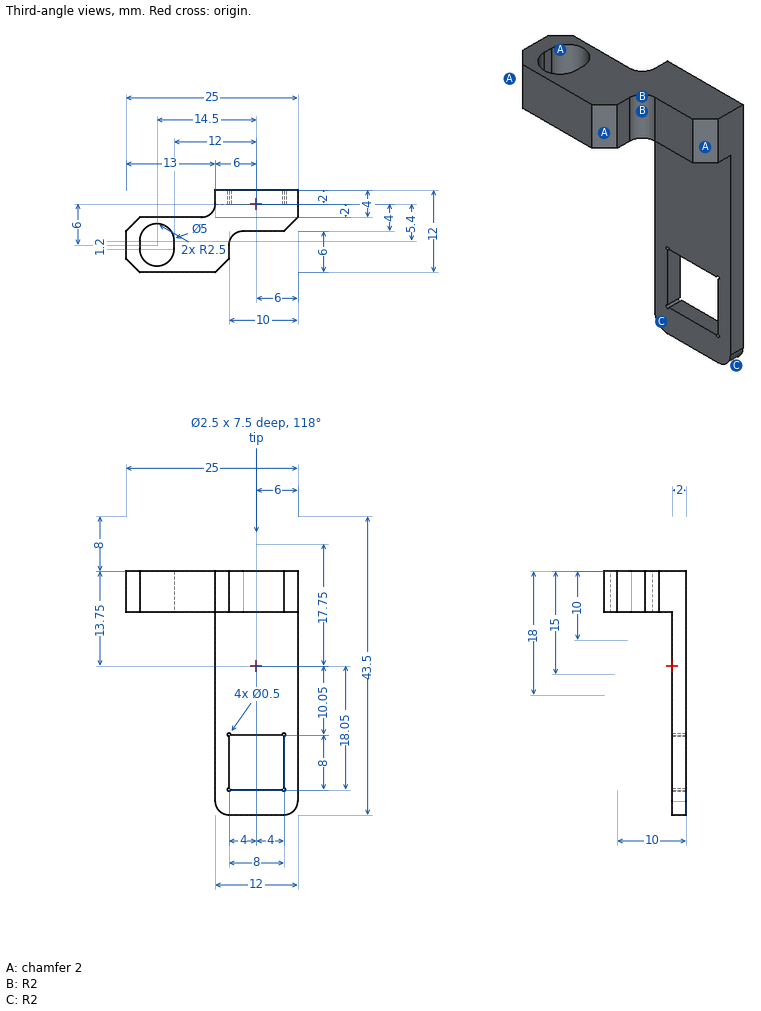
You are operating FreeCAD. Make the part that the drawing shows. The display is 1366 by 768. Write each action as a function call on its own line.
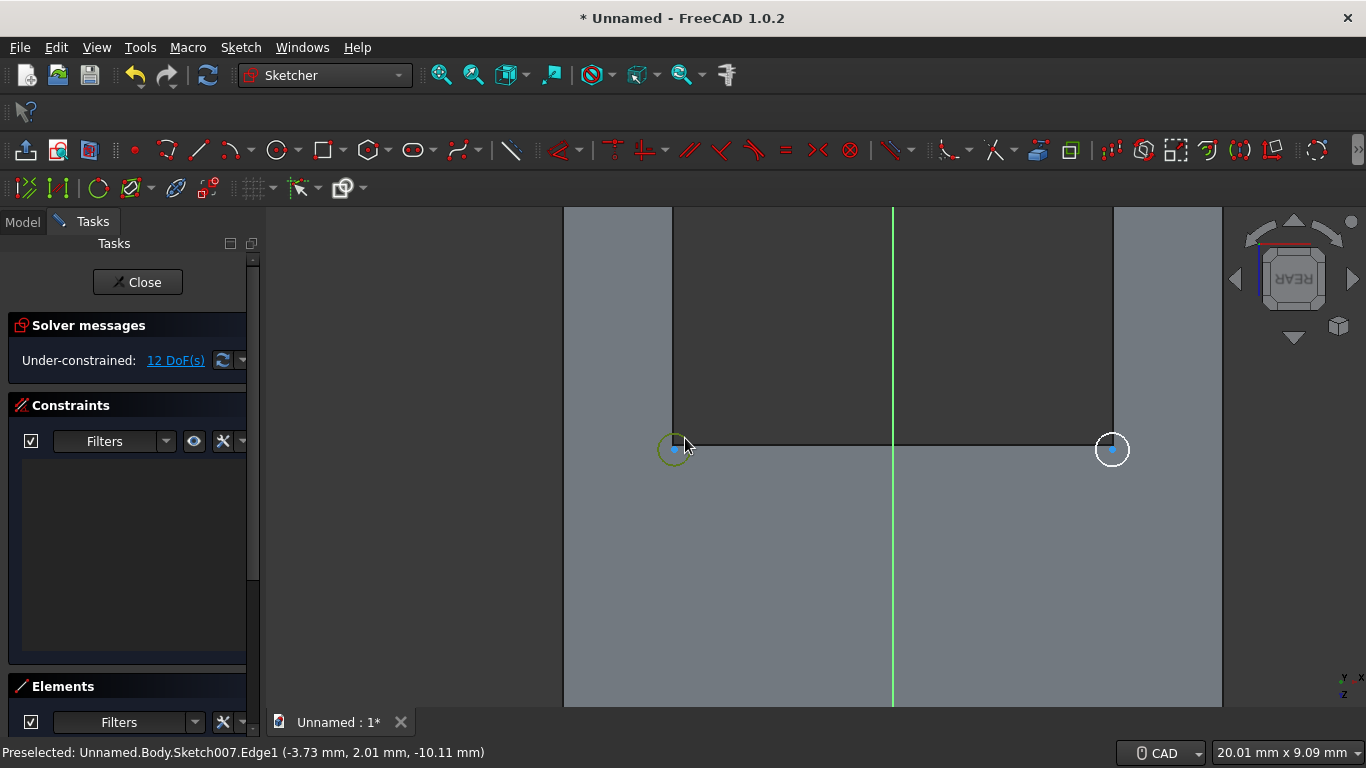
click(1124, 438)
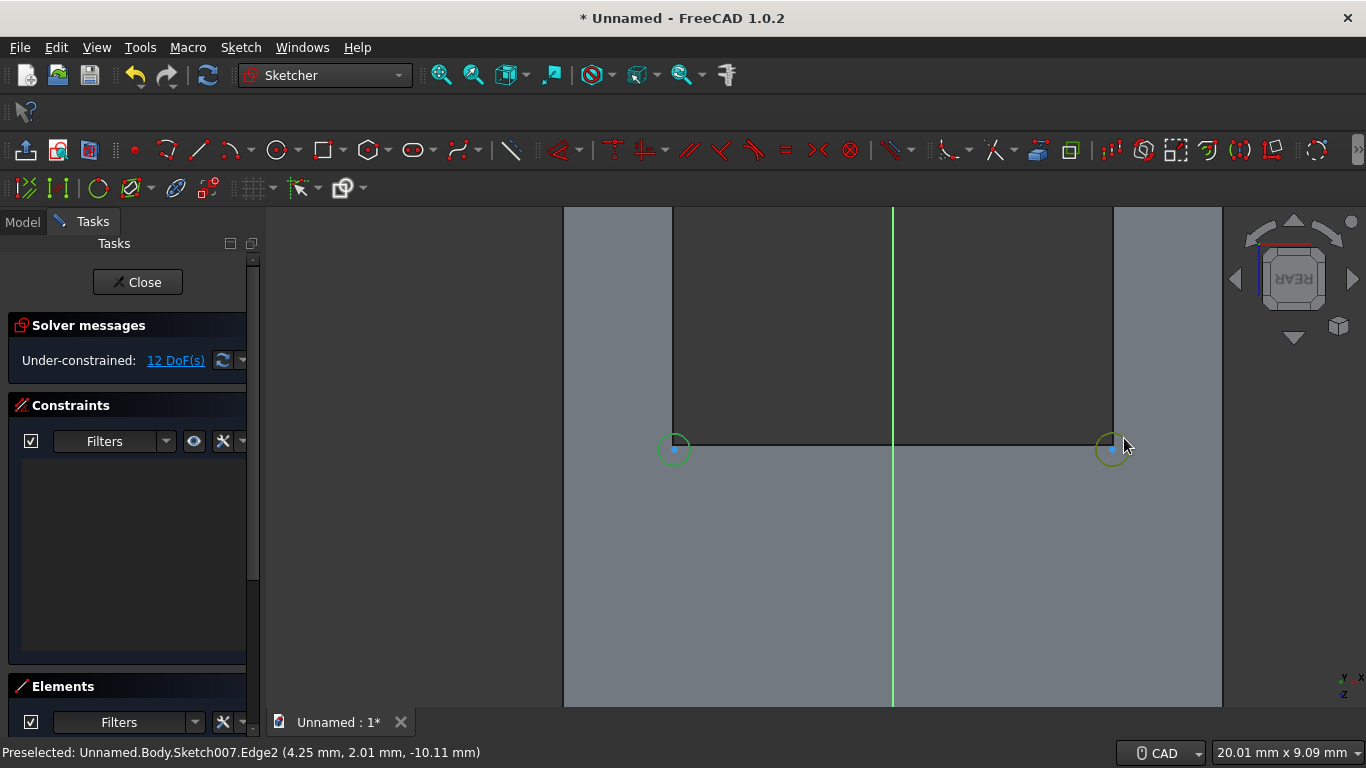
scroll(685, 441, down, 6)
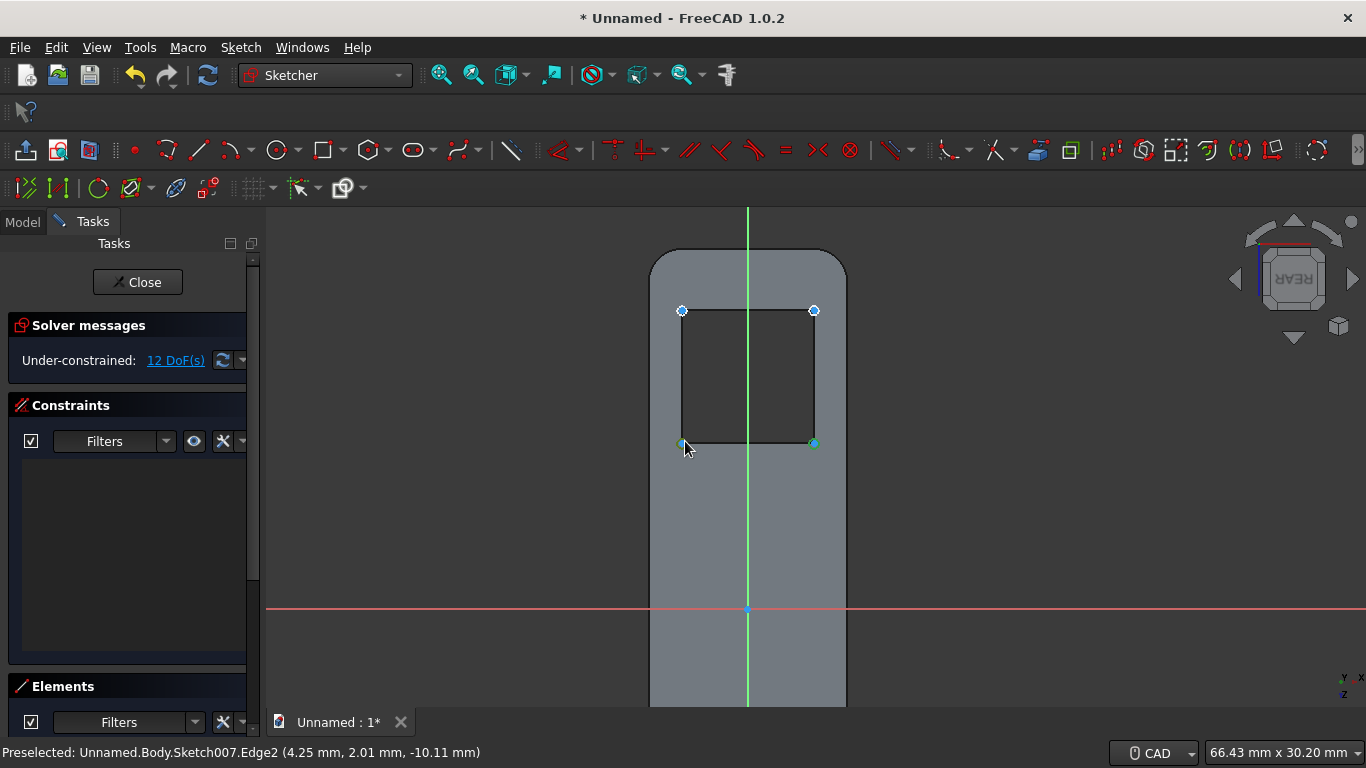
scroll(685, 308, up, 6)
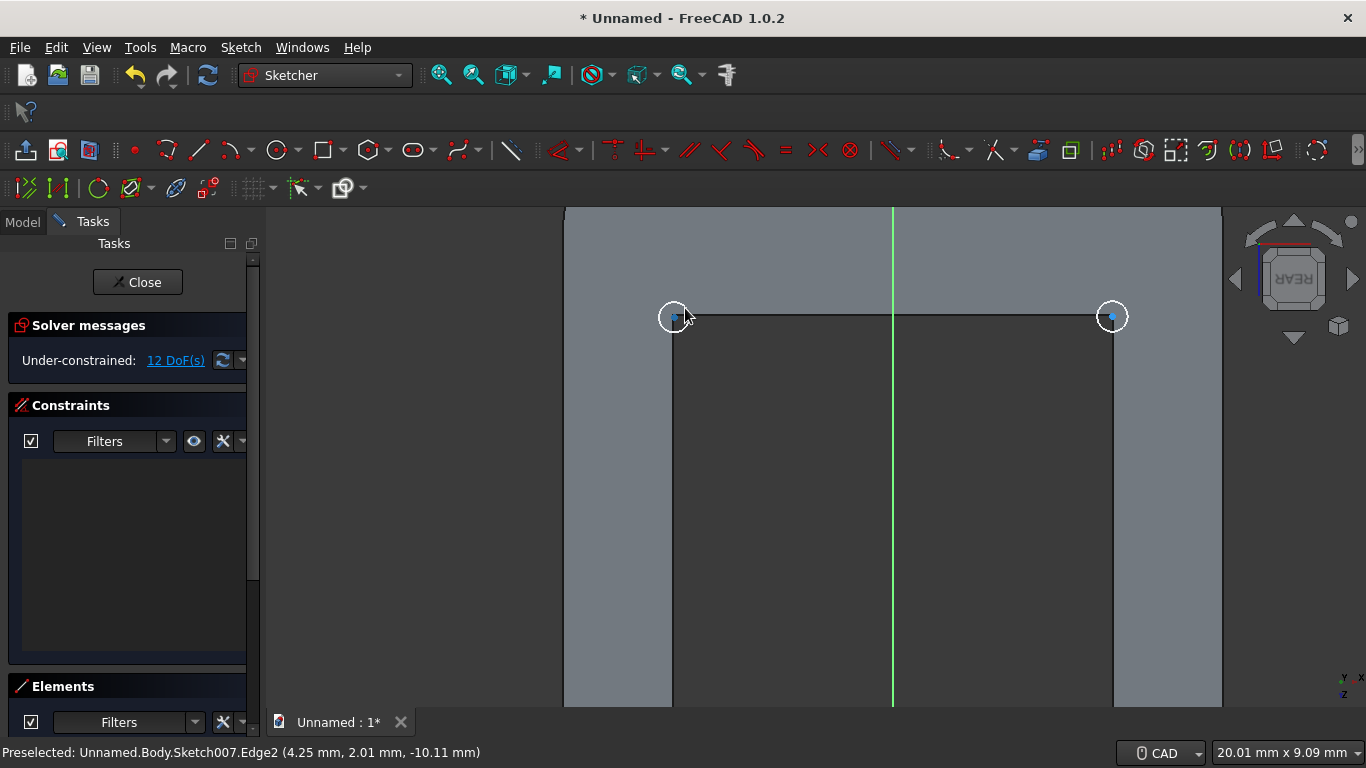
click(685, 307)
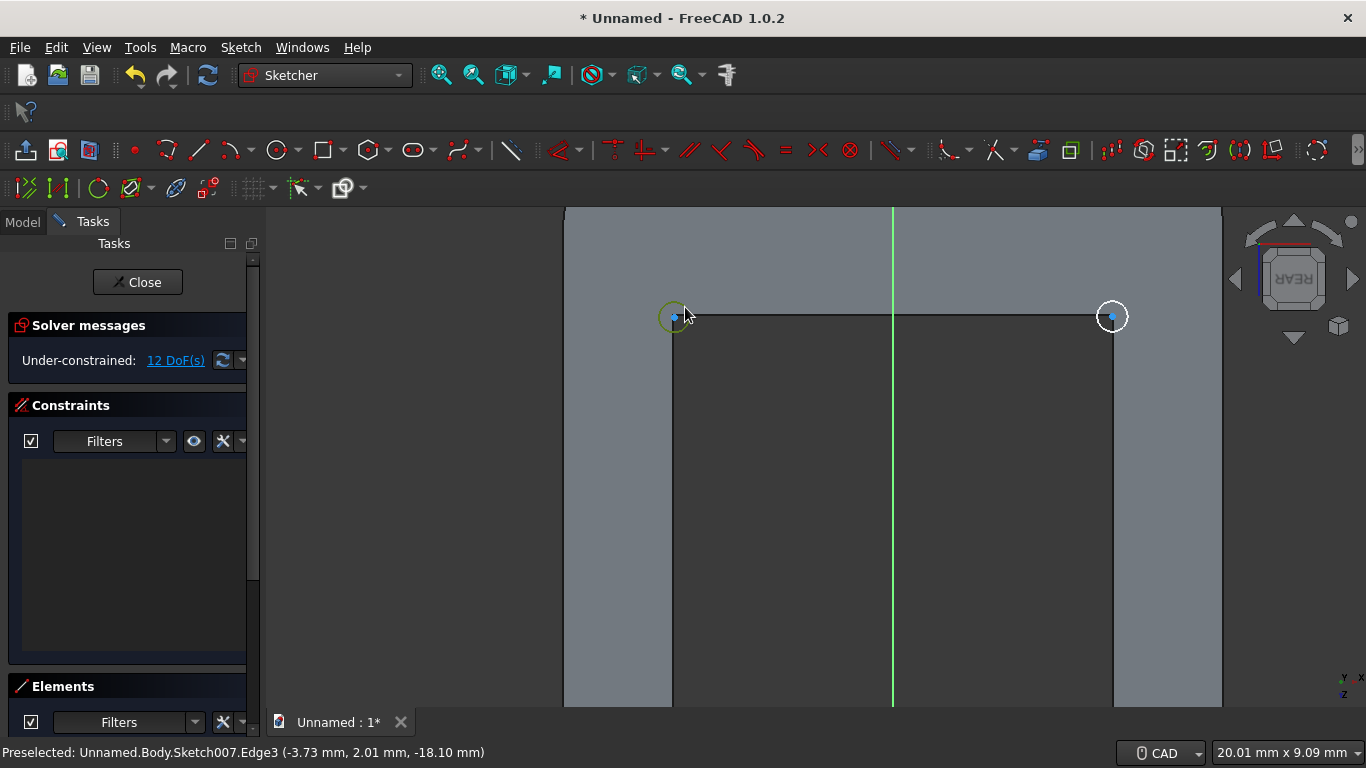
click(1123, 306)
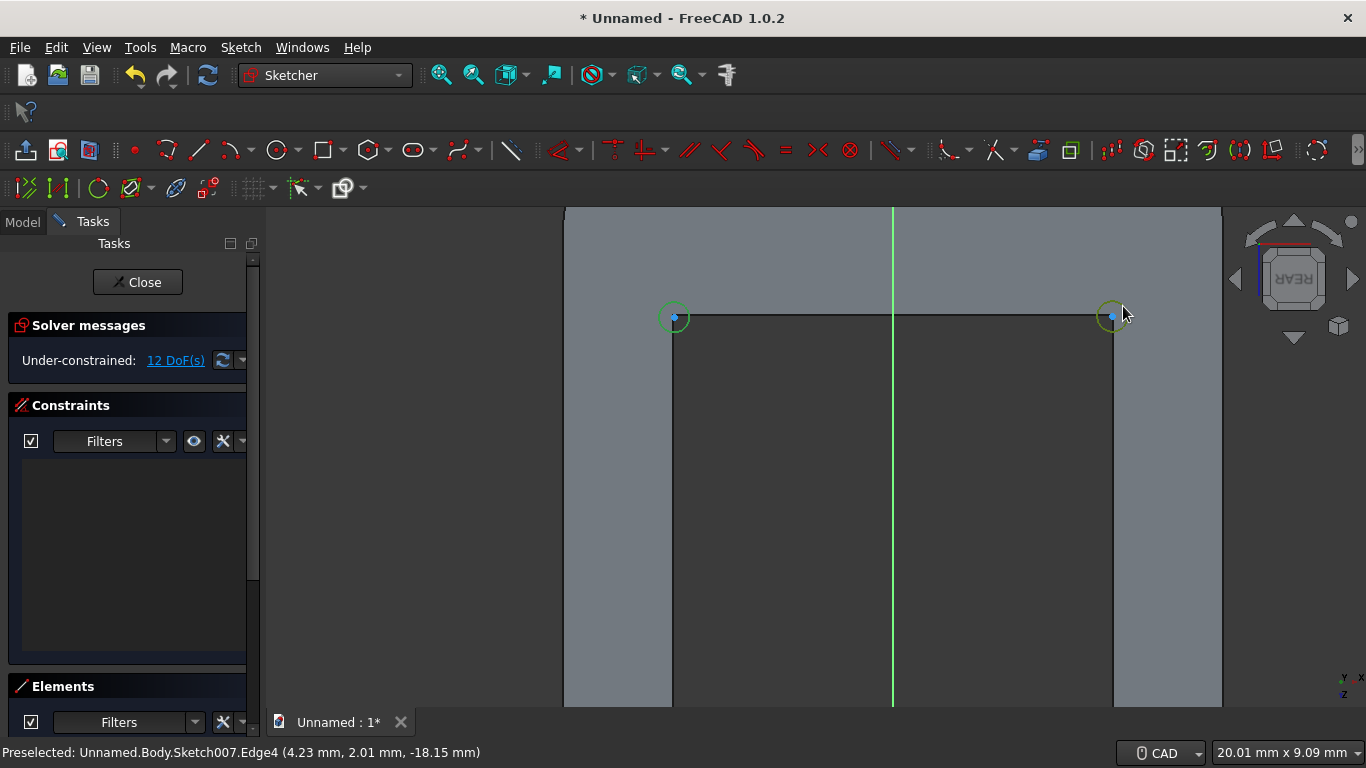
click(786, 150)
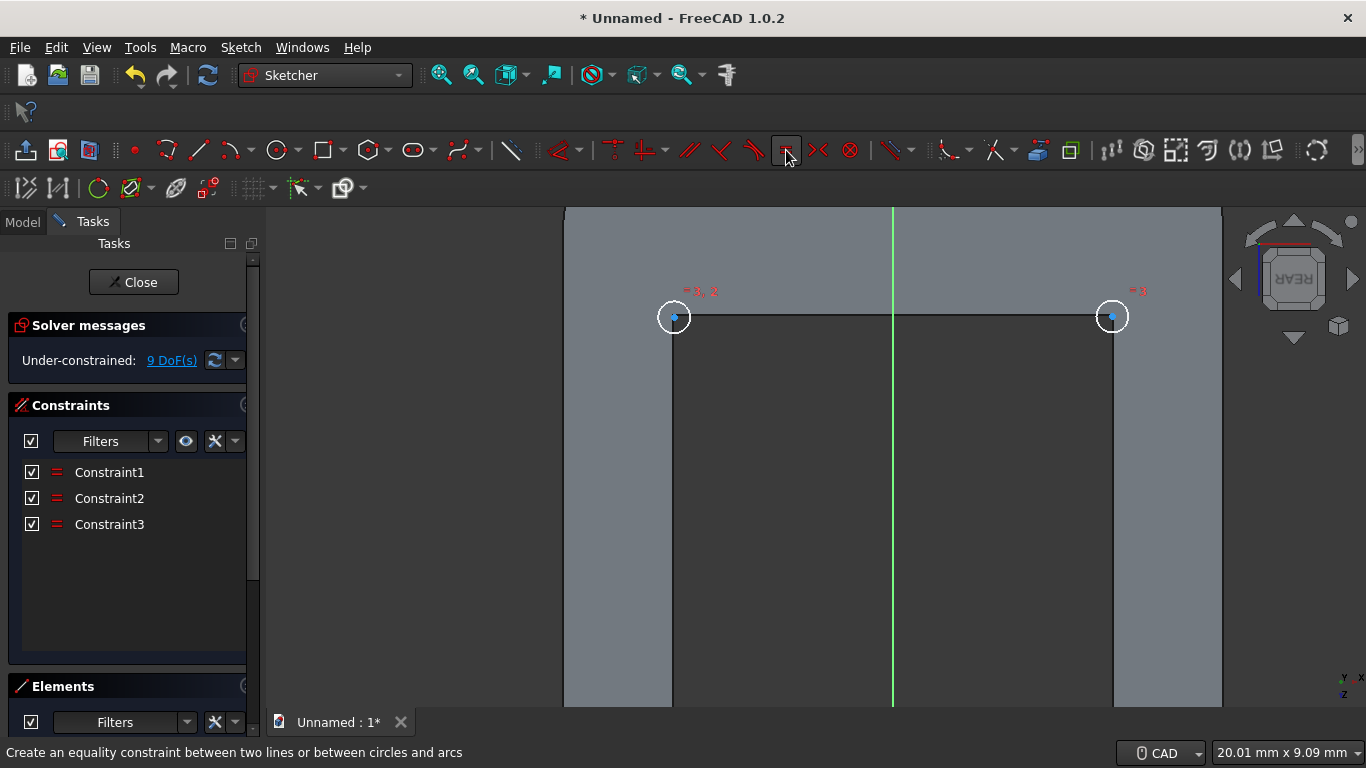
scroll(685, 307, down, 6)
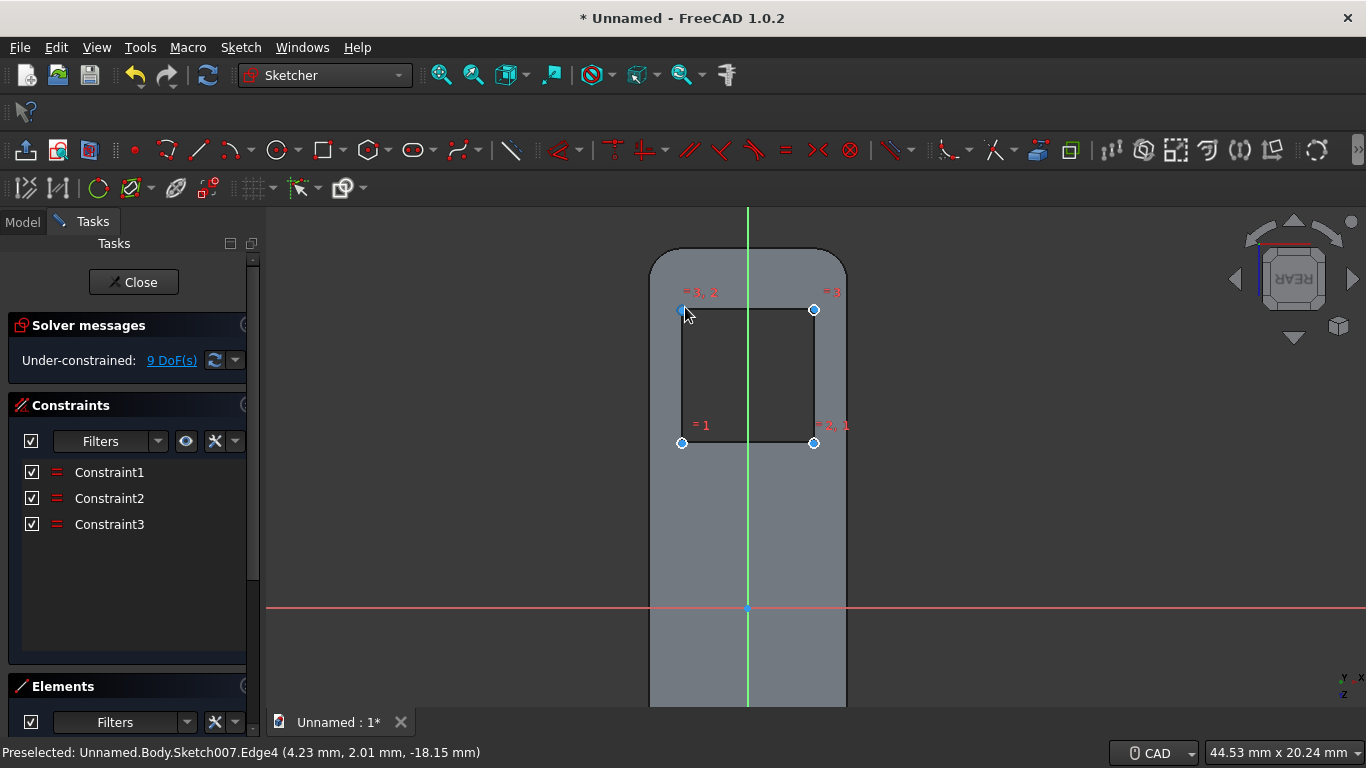
click(682, 443)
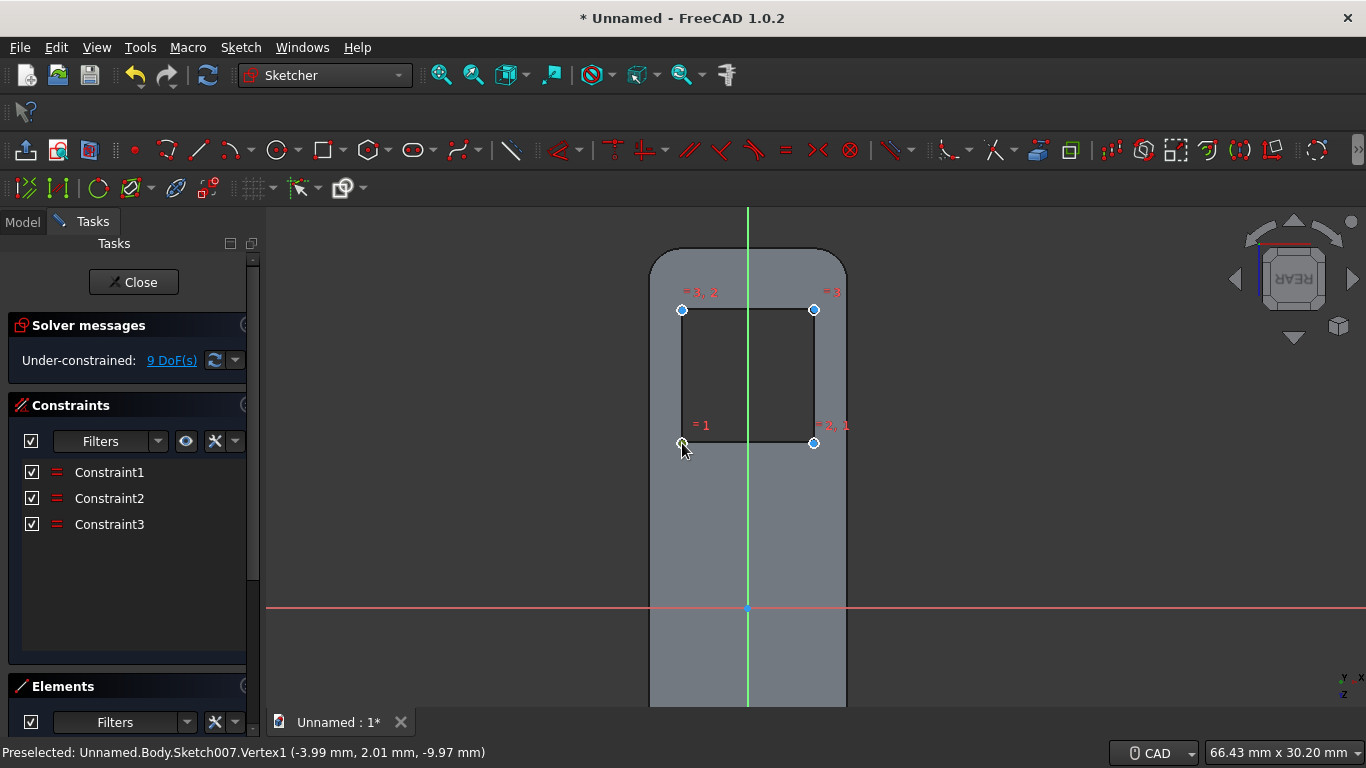
click(814, 443)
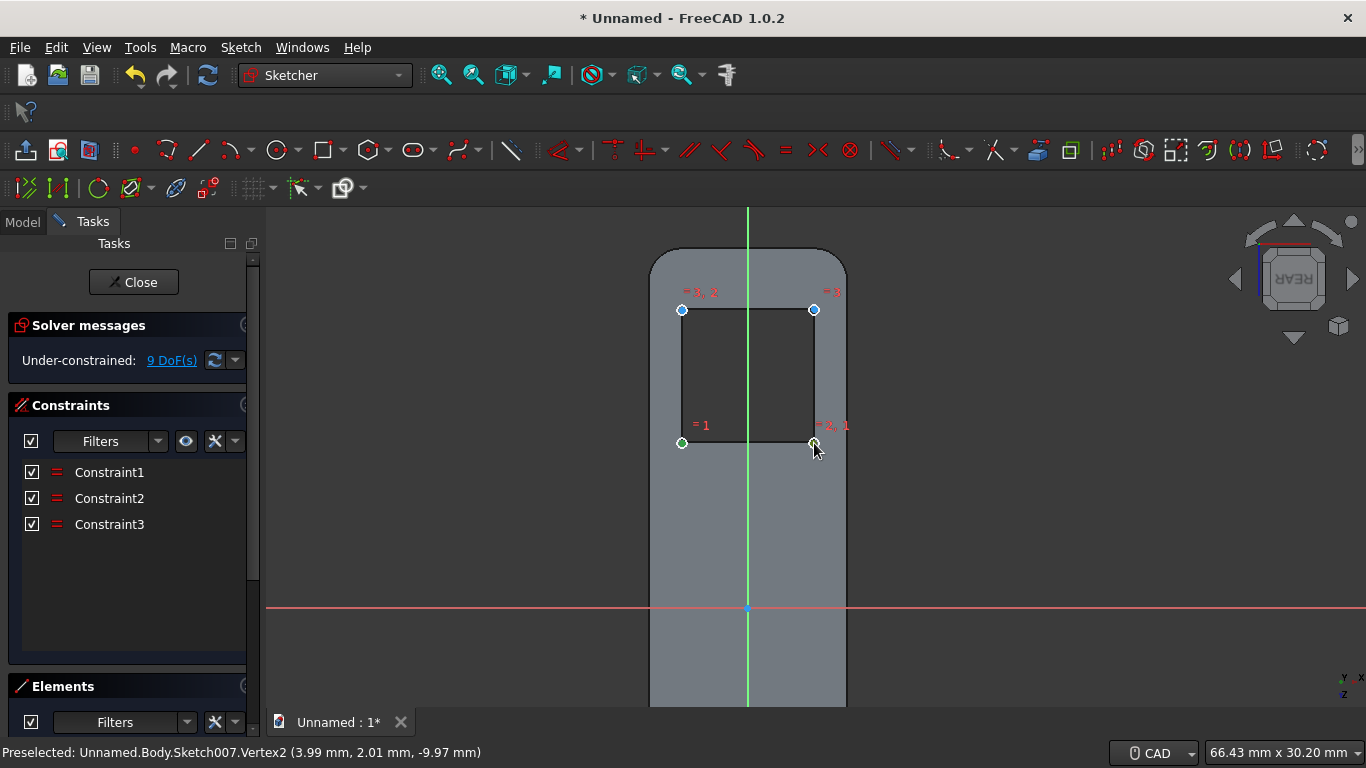
key(h)